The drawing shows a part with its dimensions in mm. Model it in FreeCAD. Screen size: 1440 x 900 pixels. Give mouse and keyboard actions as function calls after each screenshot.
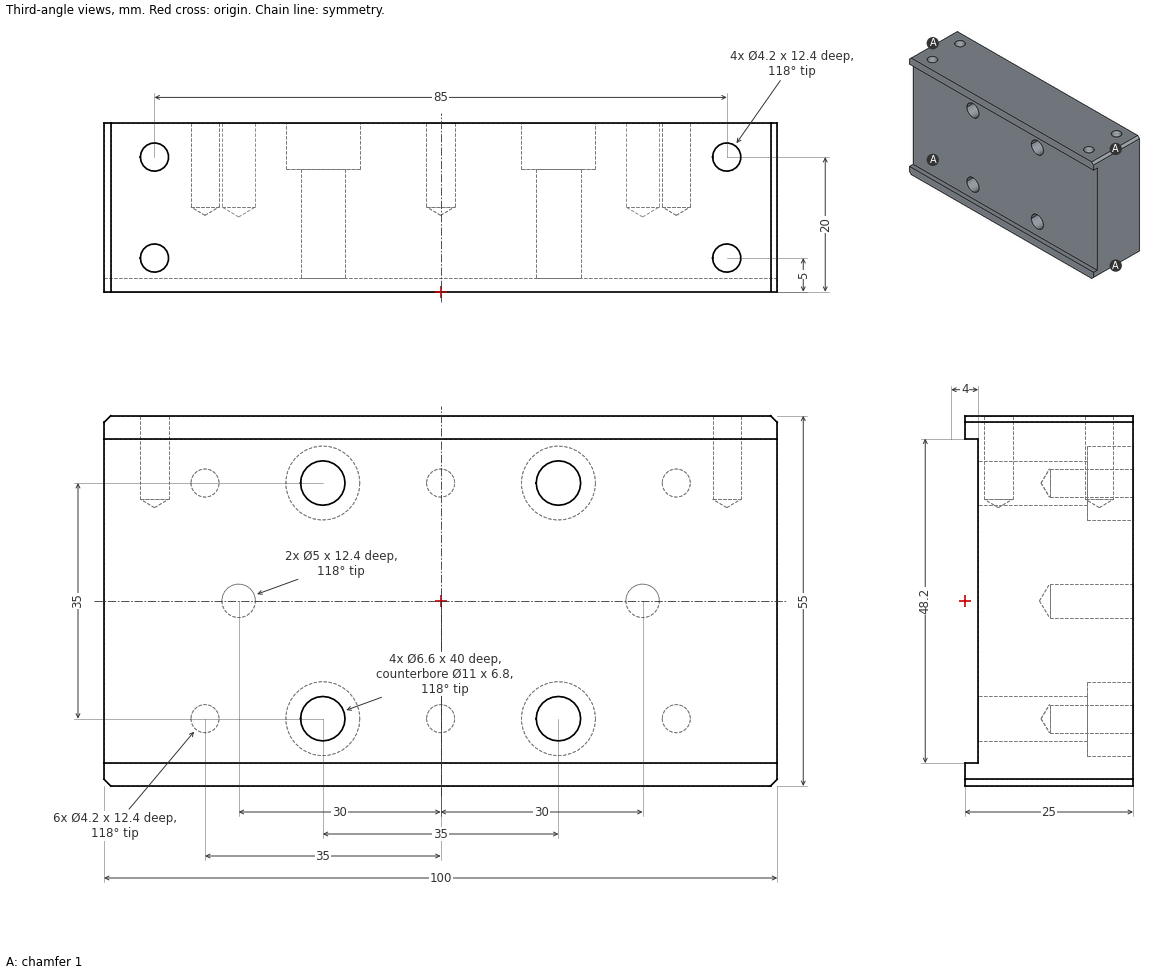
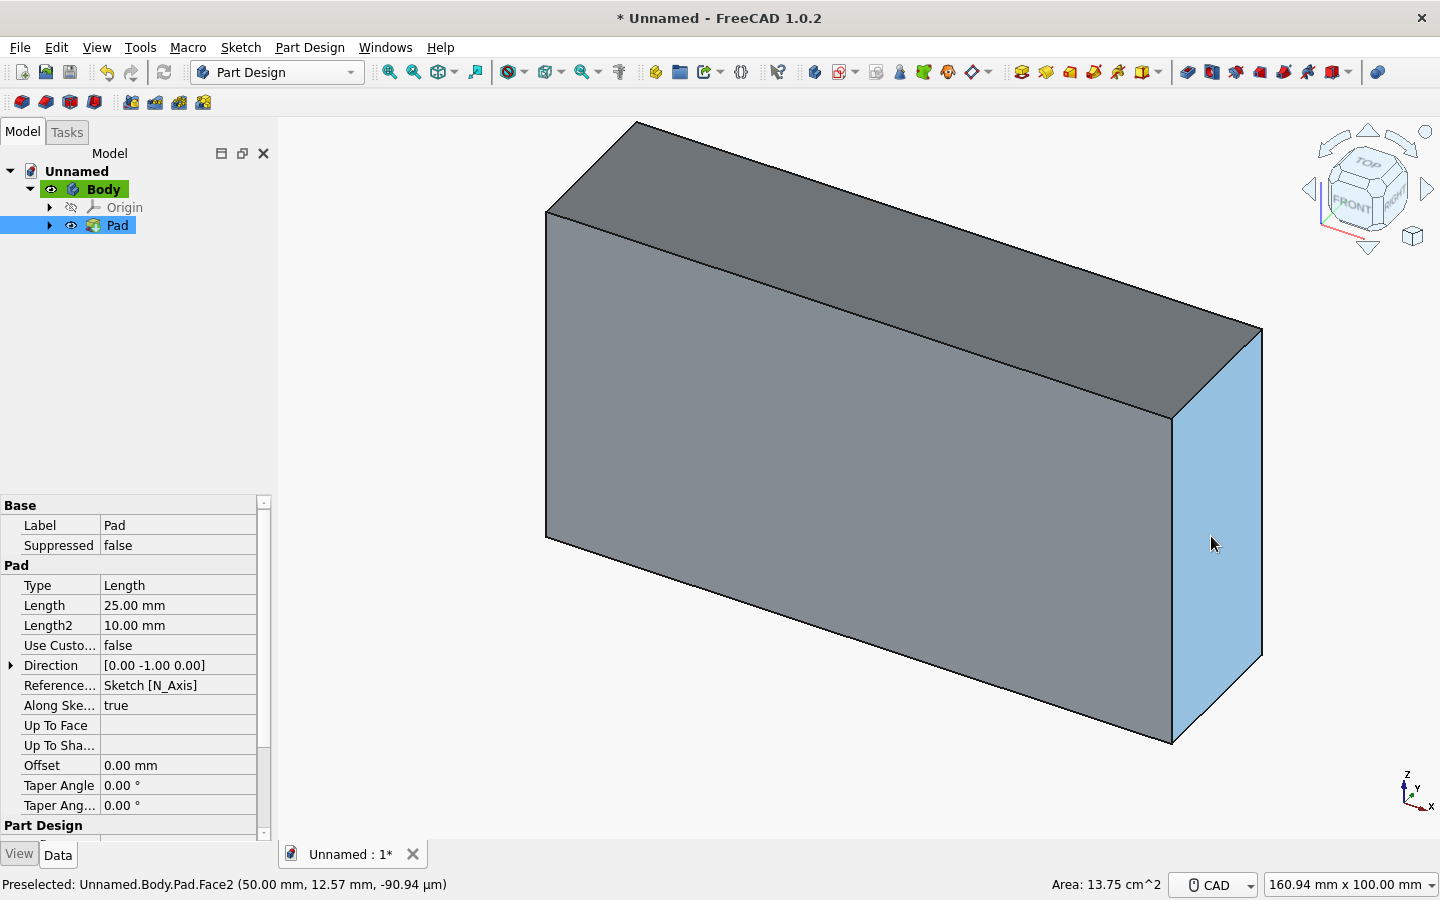
click(840, 72)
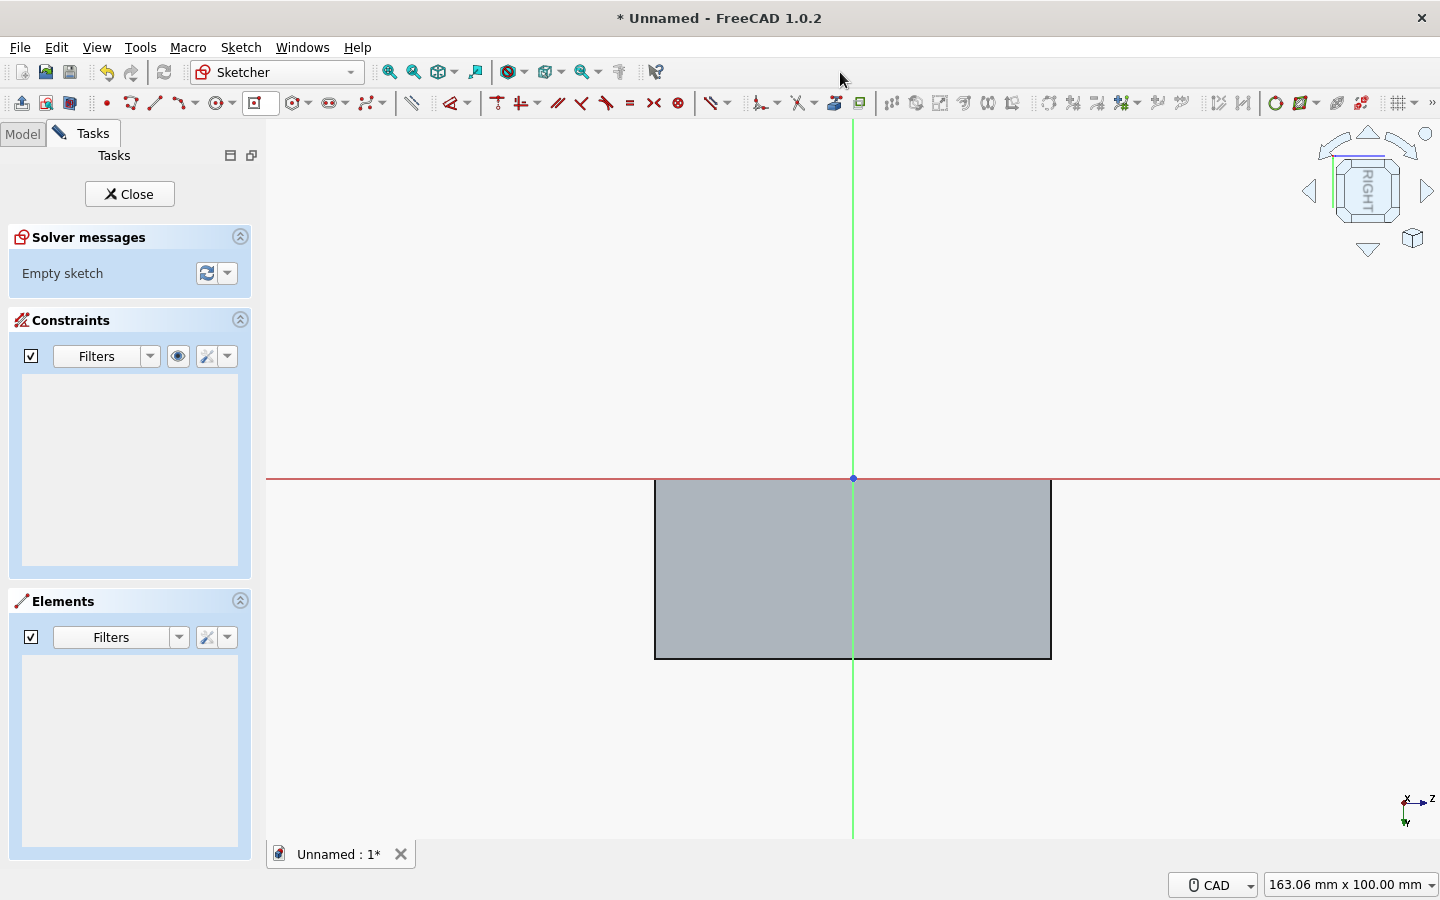
scroll(936, 479, up, 3)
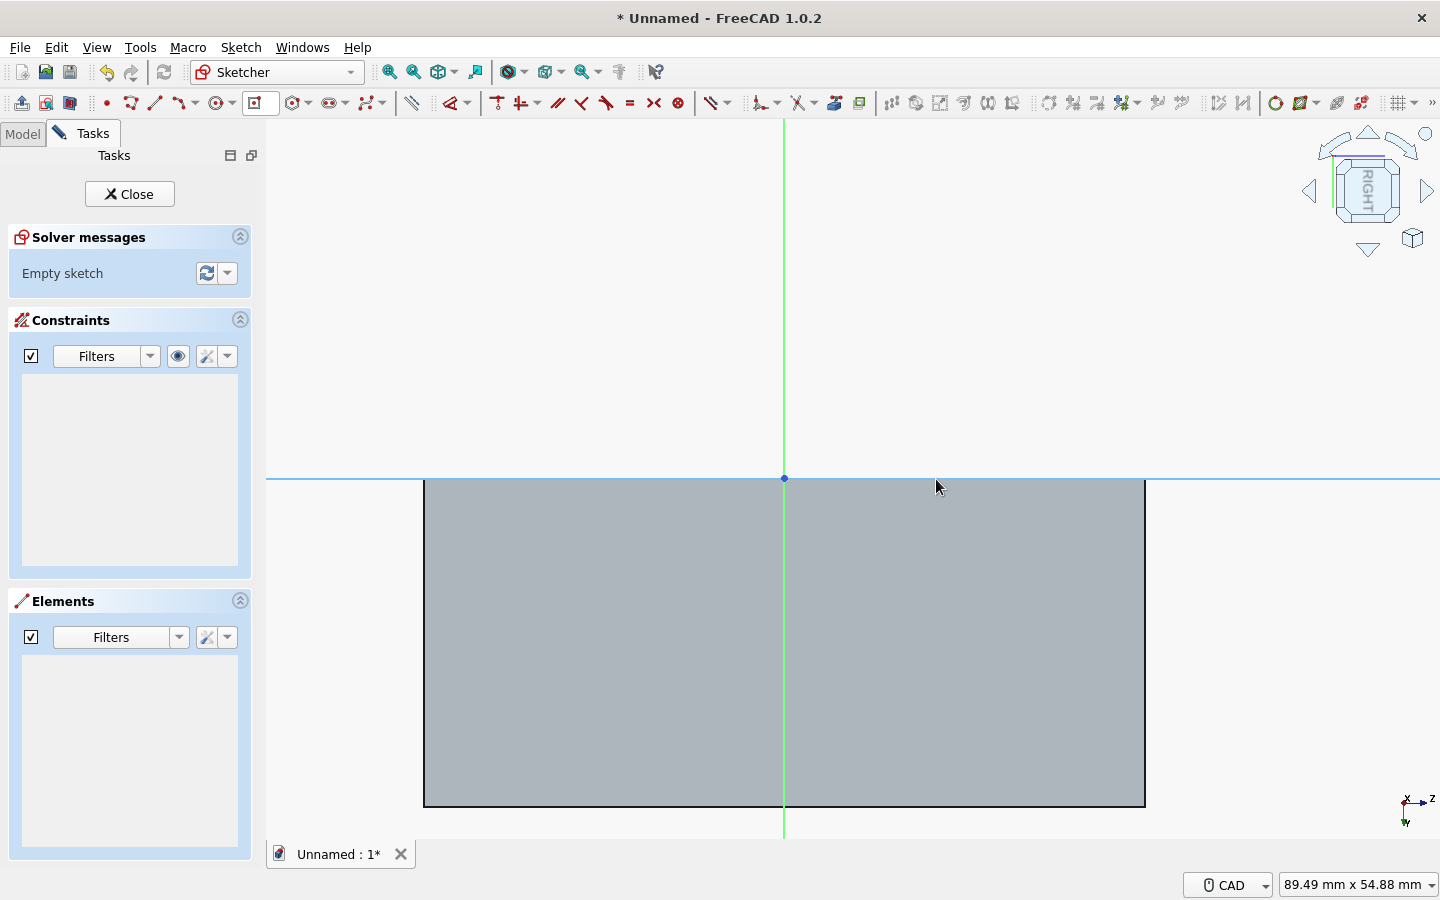
click(254, 104)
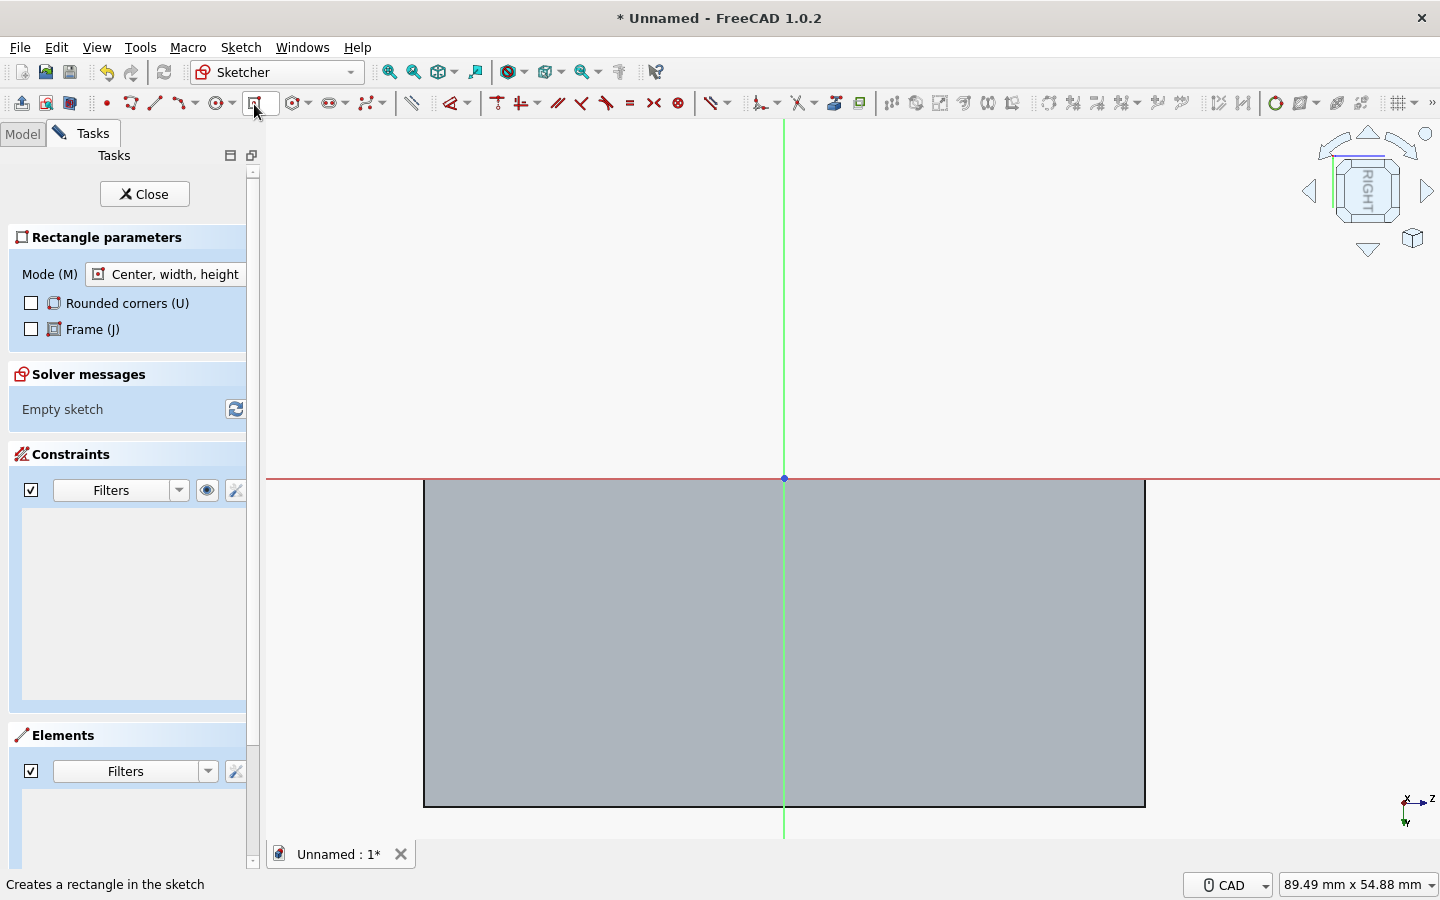
click(784, 479)
move(1100, 452)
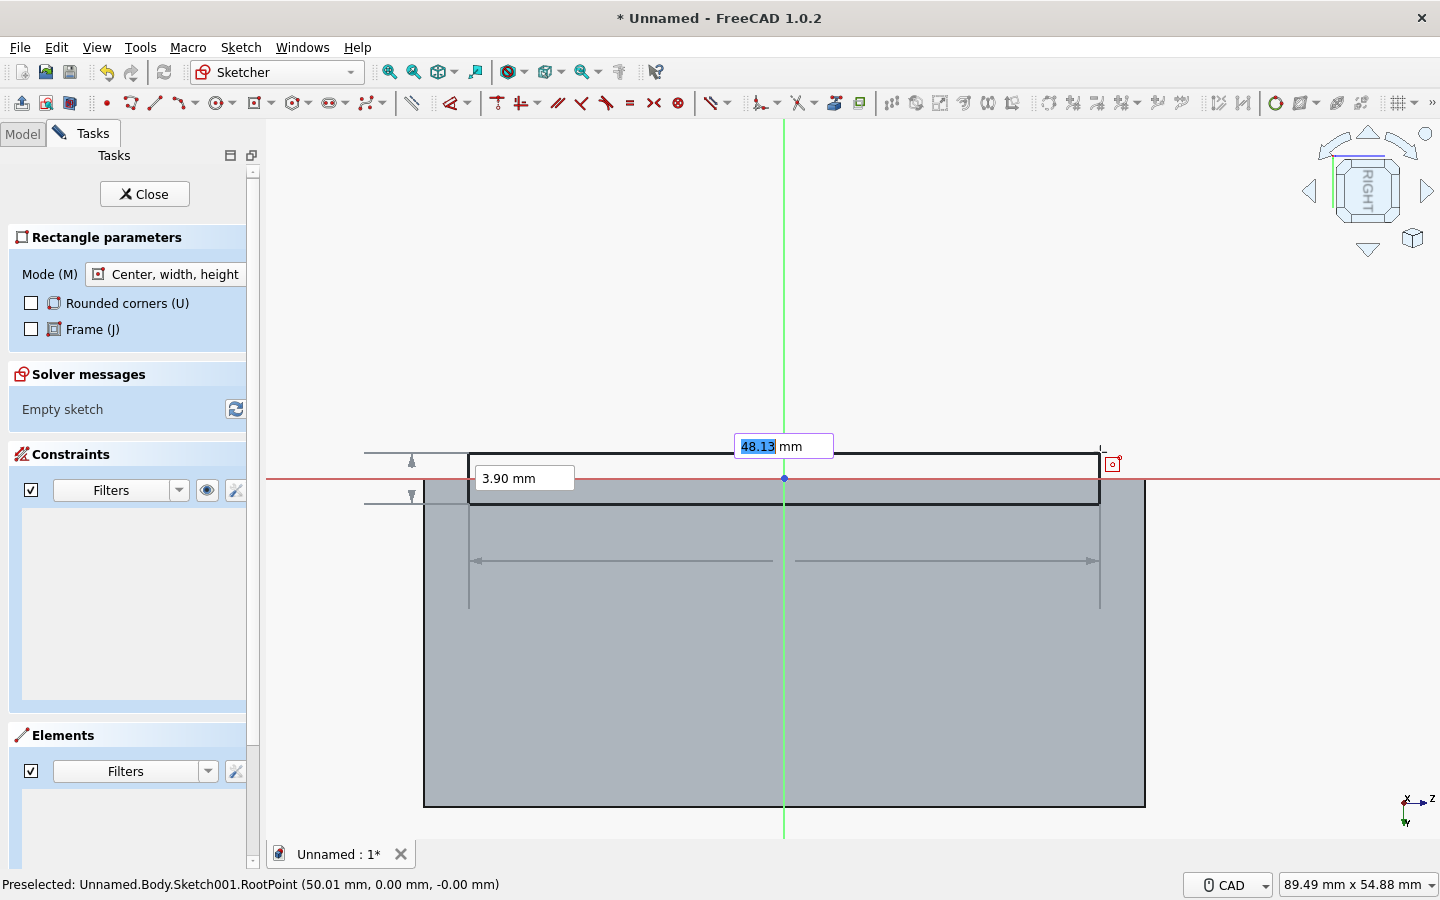
text(48.2)
key(Tab)
text(4)
key(Return)
key(Escape)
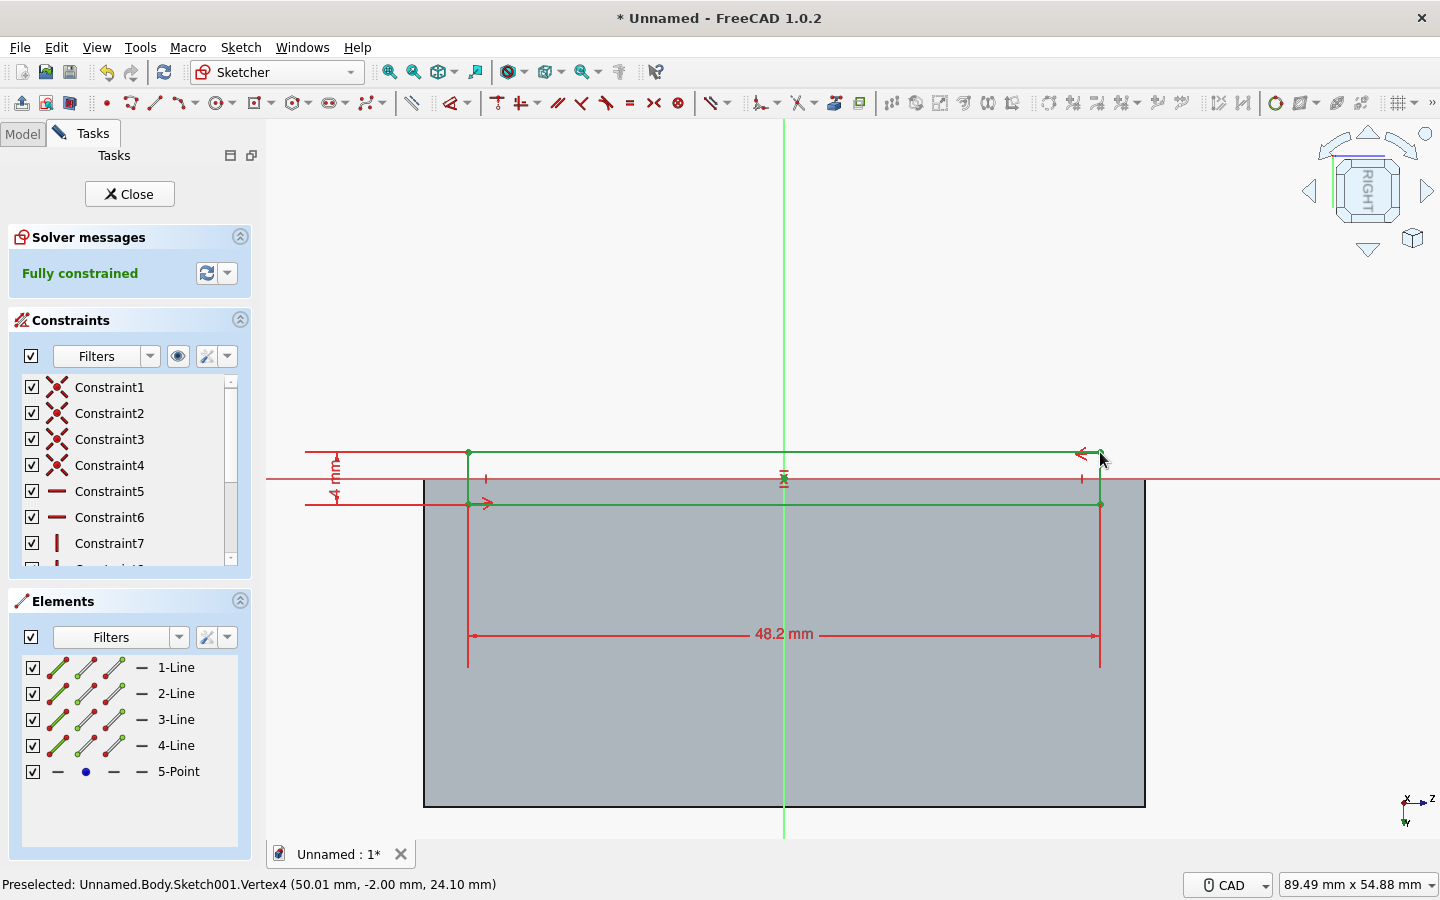
click(130, 194)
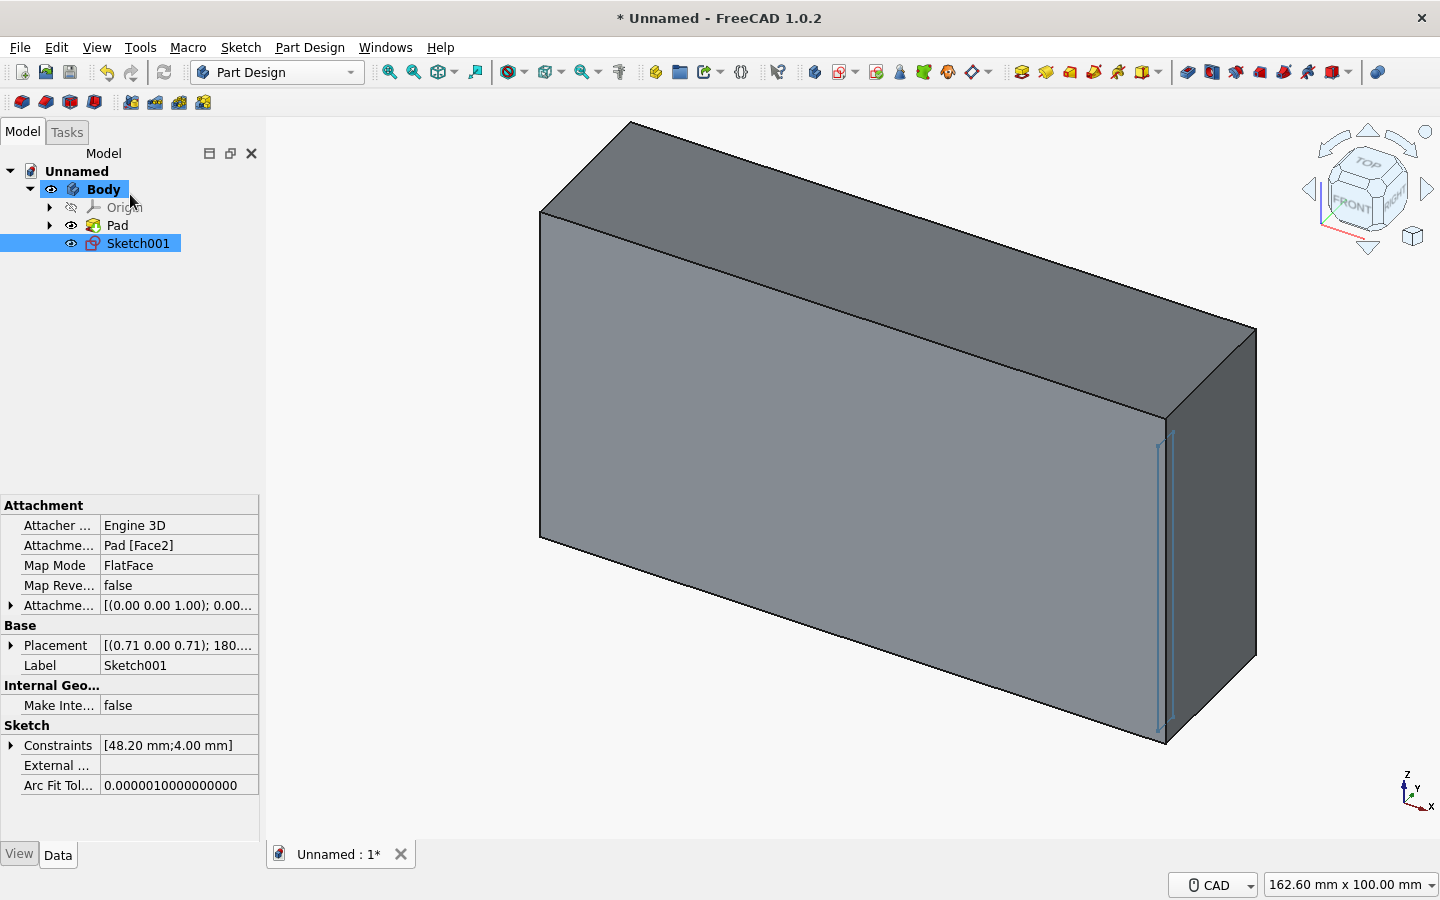
click(1188, 72)